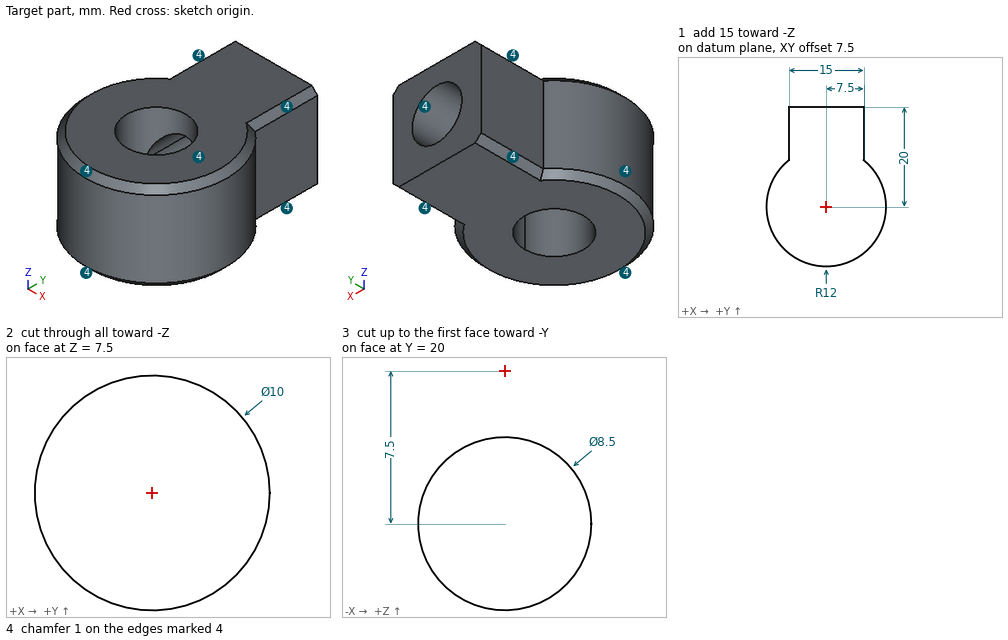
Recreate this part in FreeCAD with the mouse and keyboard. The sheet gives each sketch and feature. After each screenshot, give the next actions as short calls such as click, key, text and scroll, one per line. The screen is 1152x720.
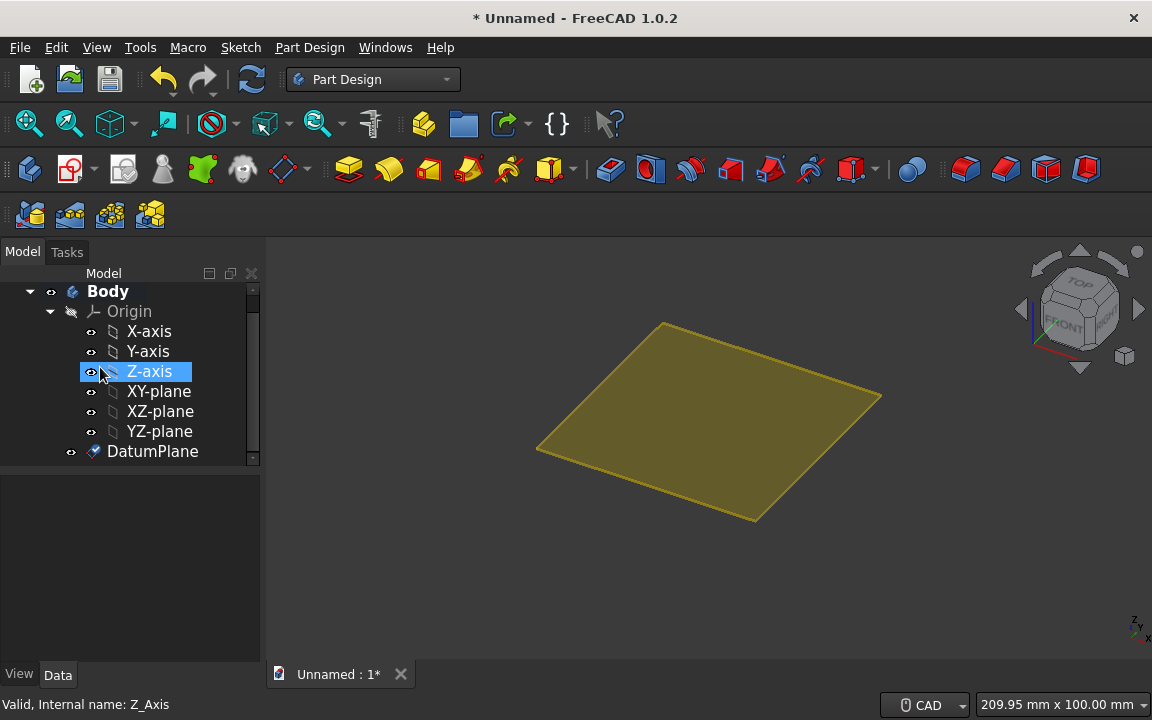
click(116, 452)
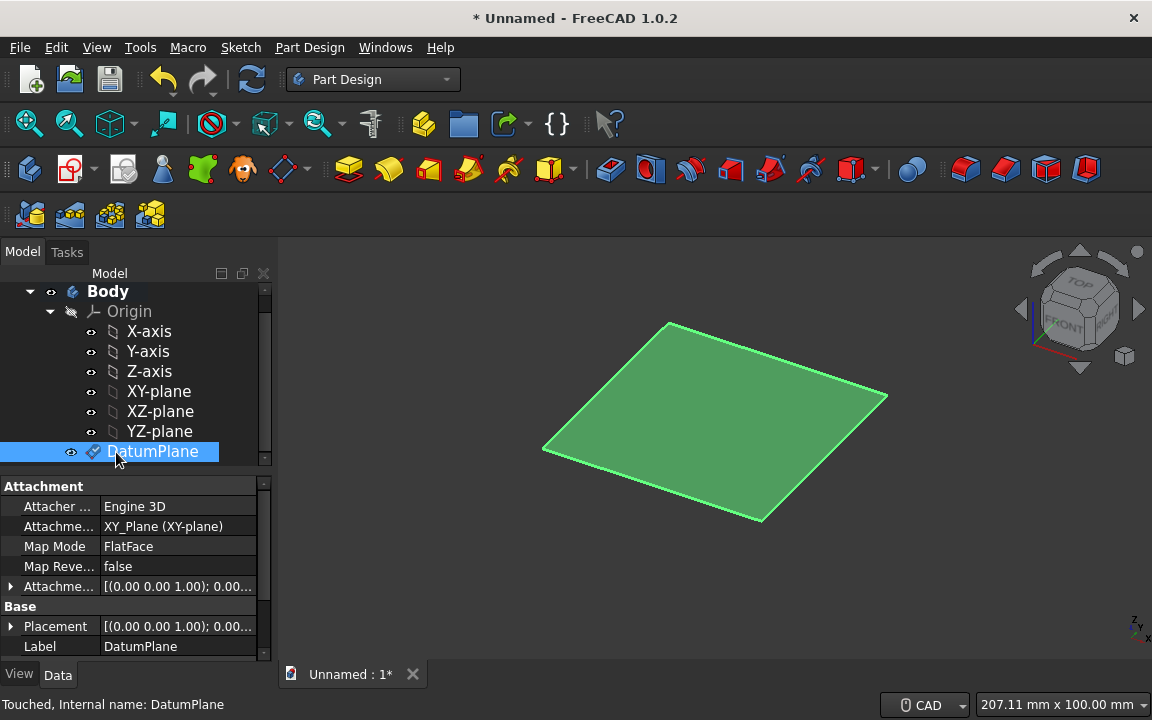
click(70, 170)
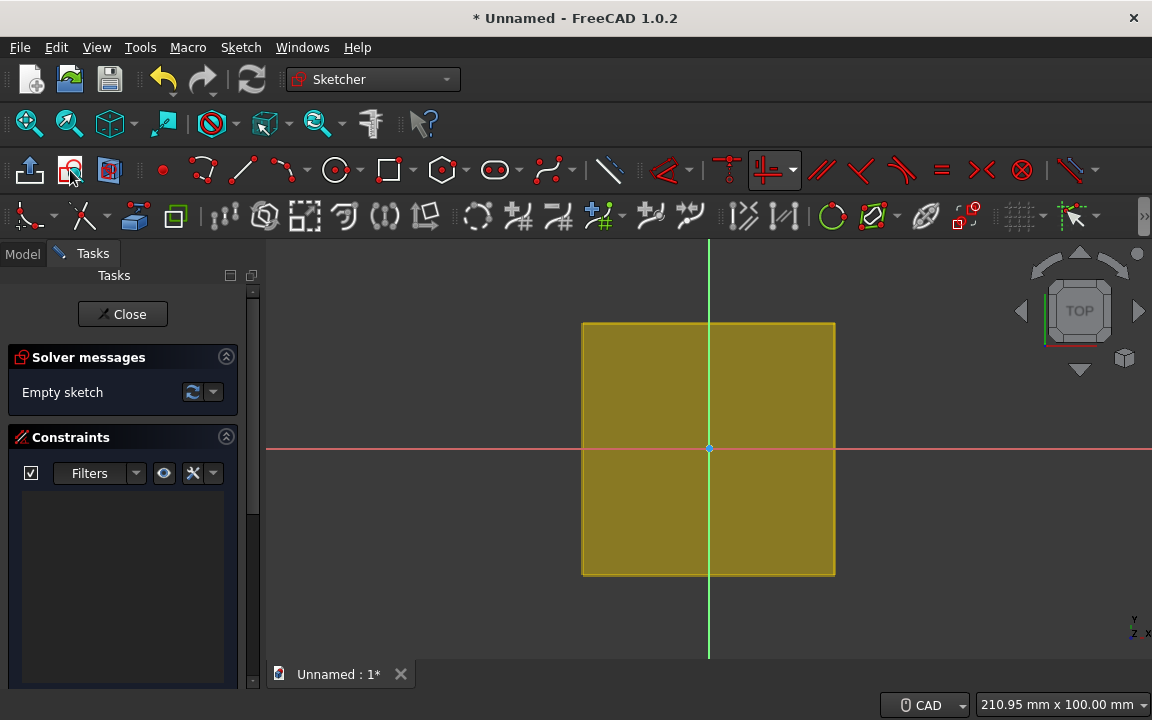
scroll(792, 412, up, 3)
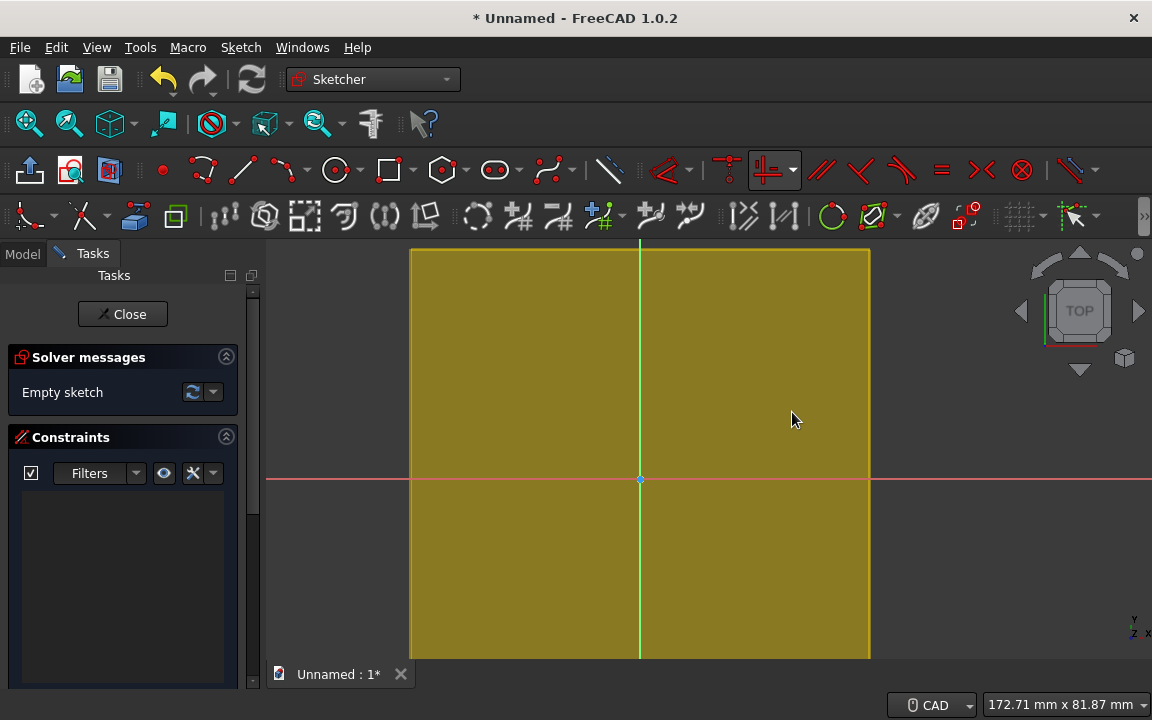
click(204, 170)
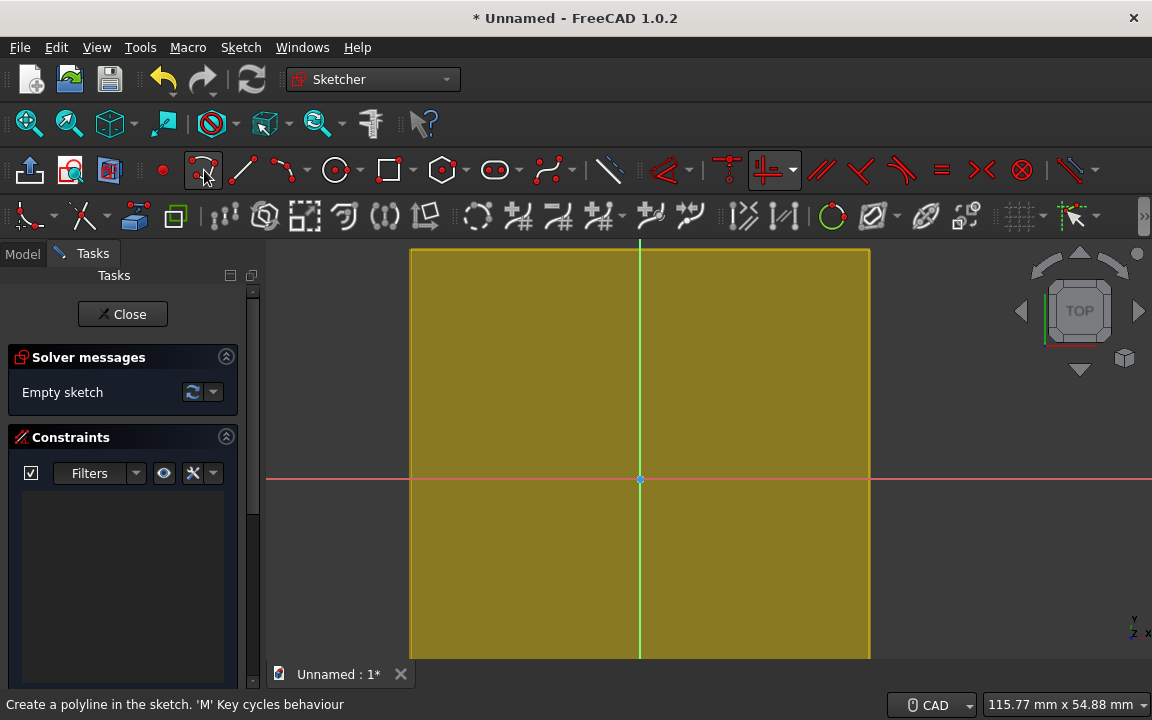
click(698, 407)
click(698, 326)
click(583, 326)
click(583, 407)
right_click(583, 407)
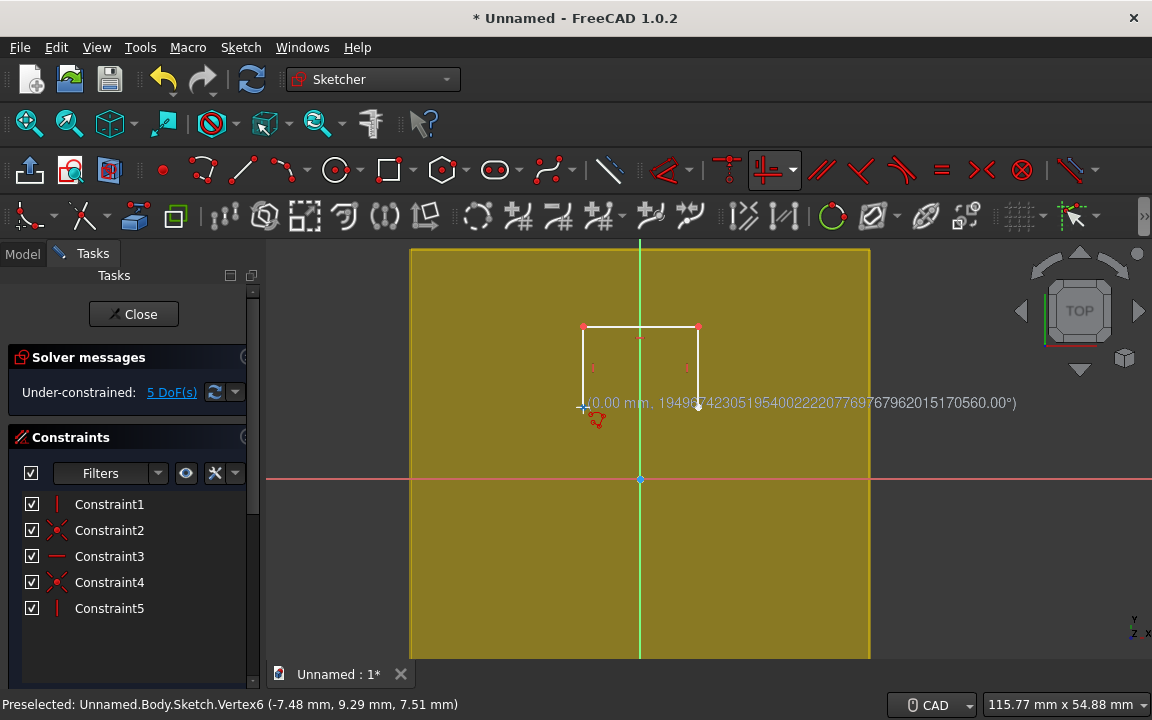
click(284, 170)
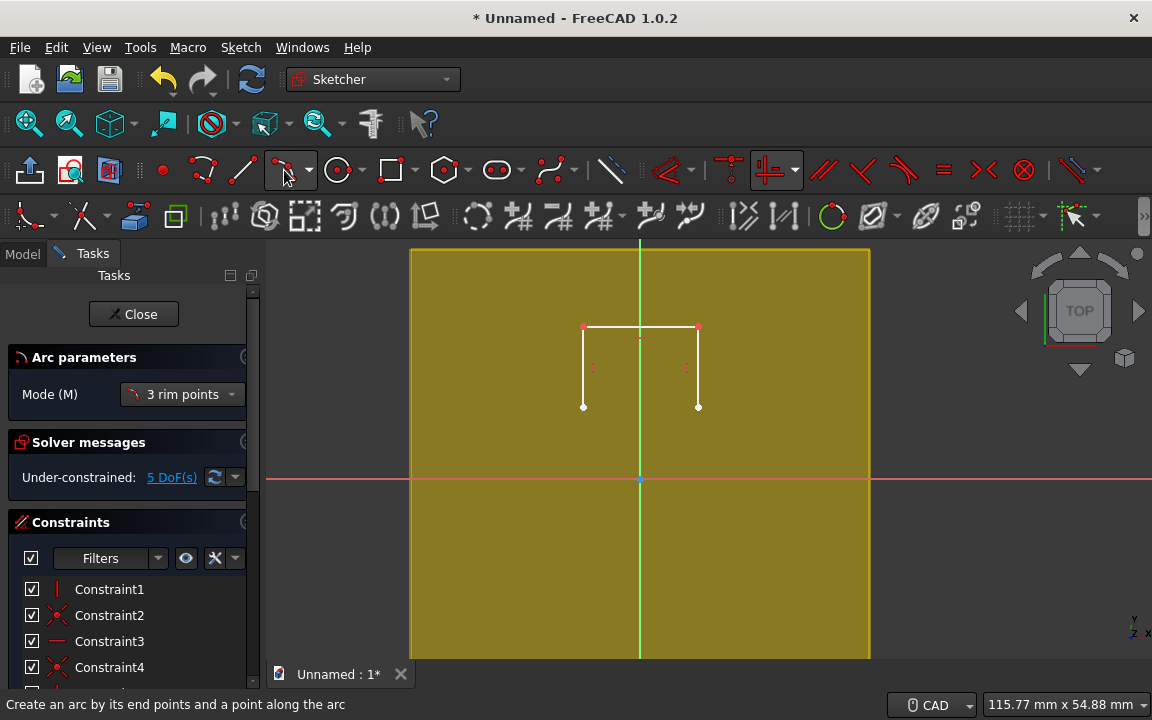
click(583, 408)
click(698, 408)
click(597, 560)
key(Escape)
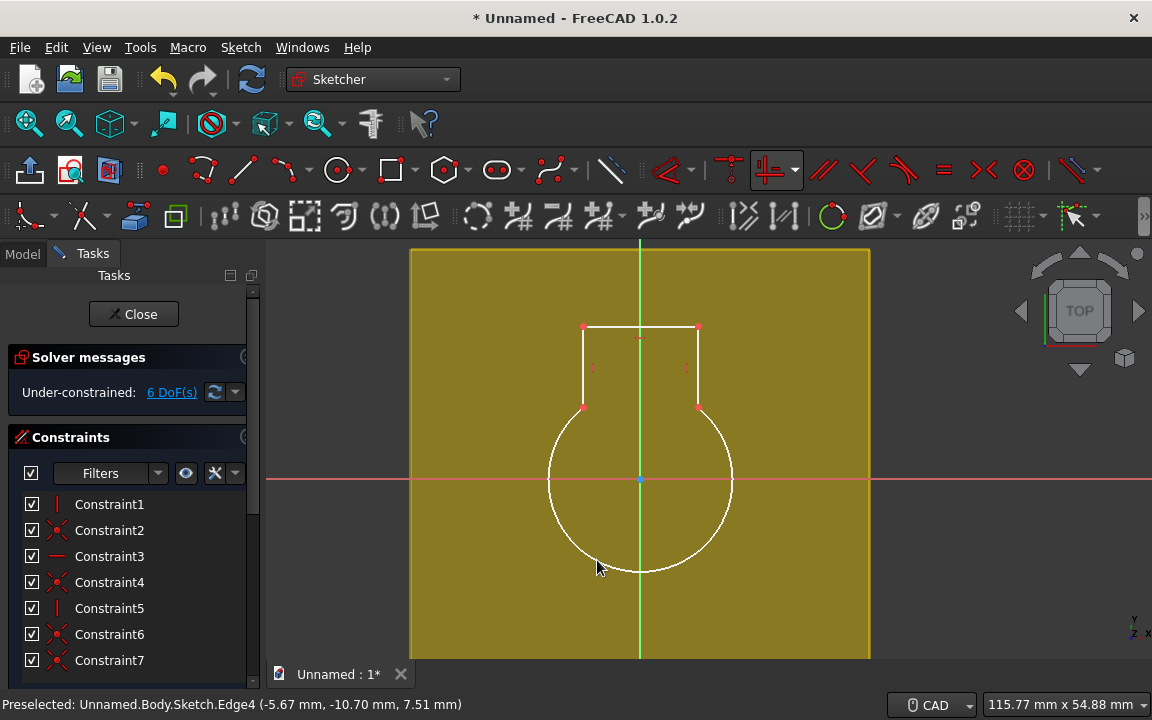
drag(630, 469, 651, 490)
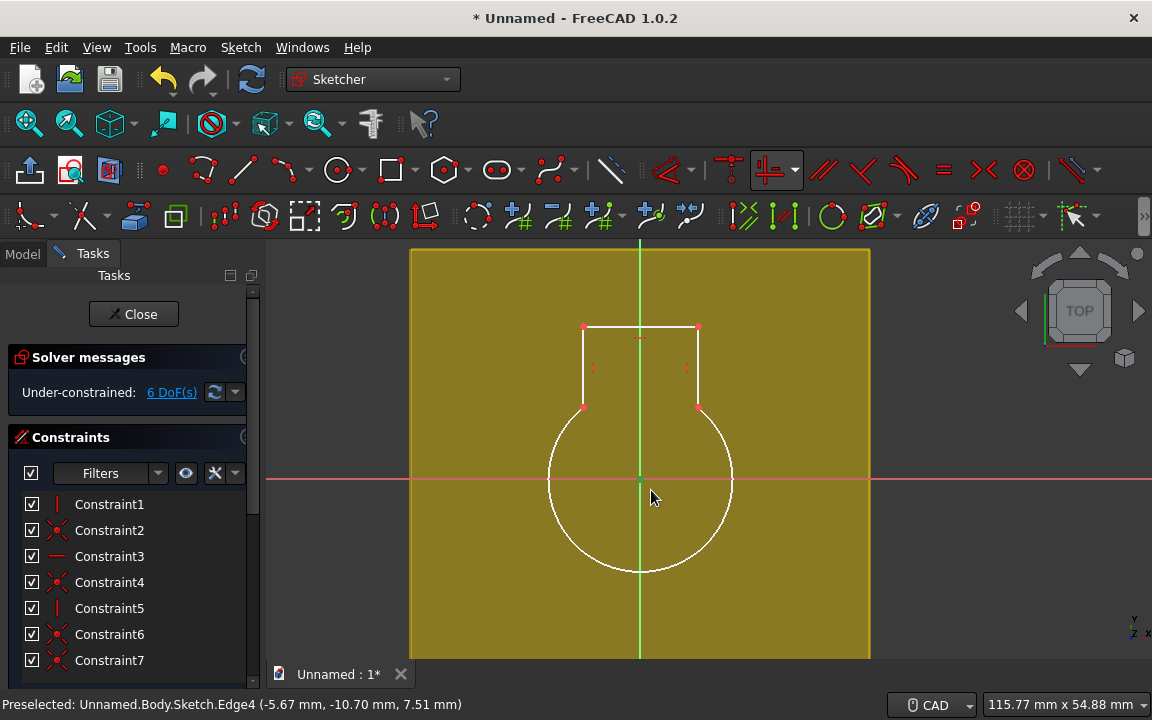
click(730, 170)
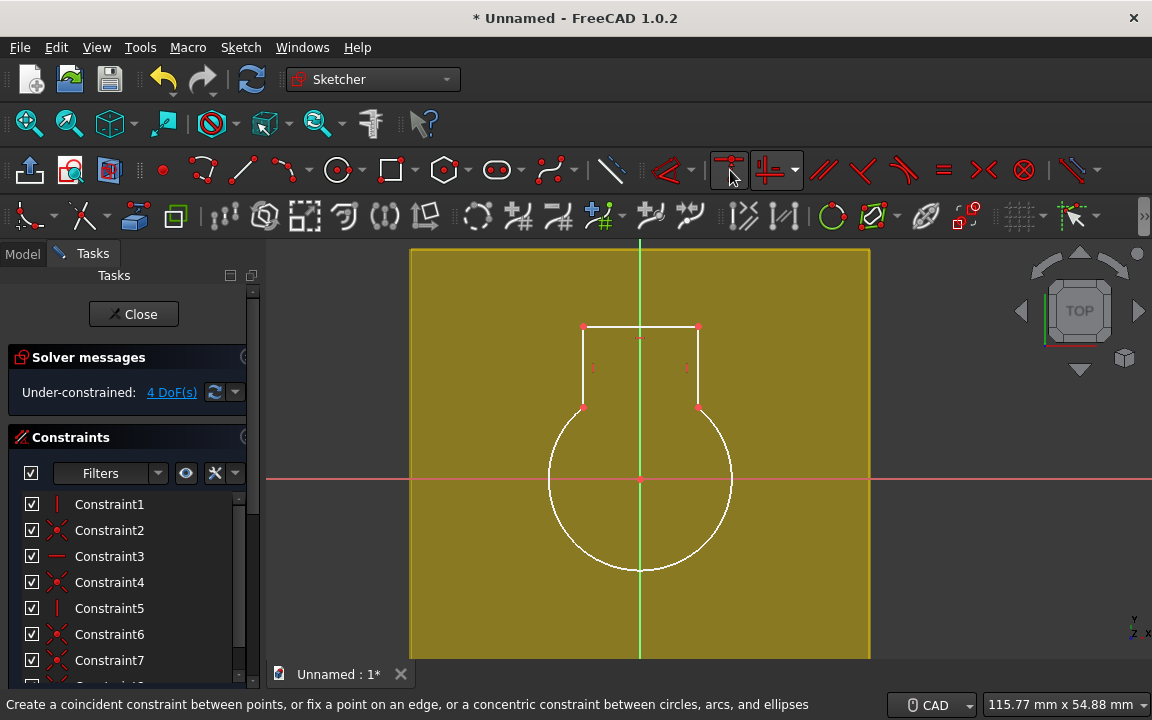
click(666, 170)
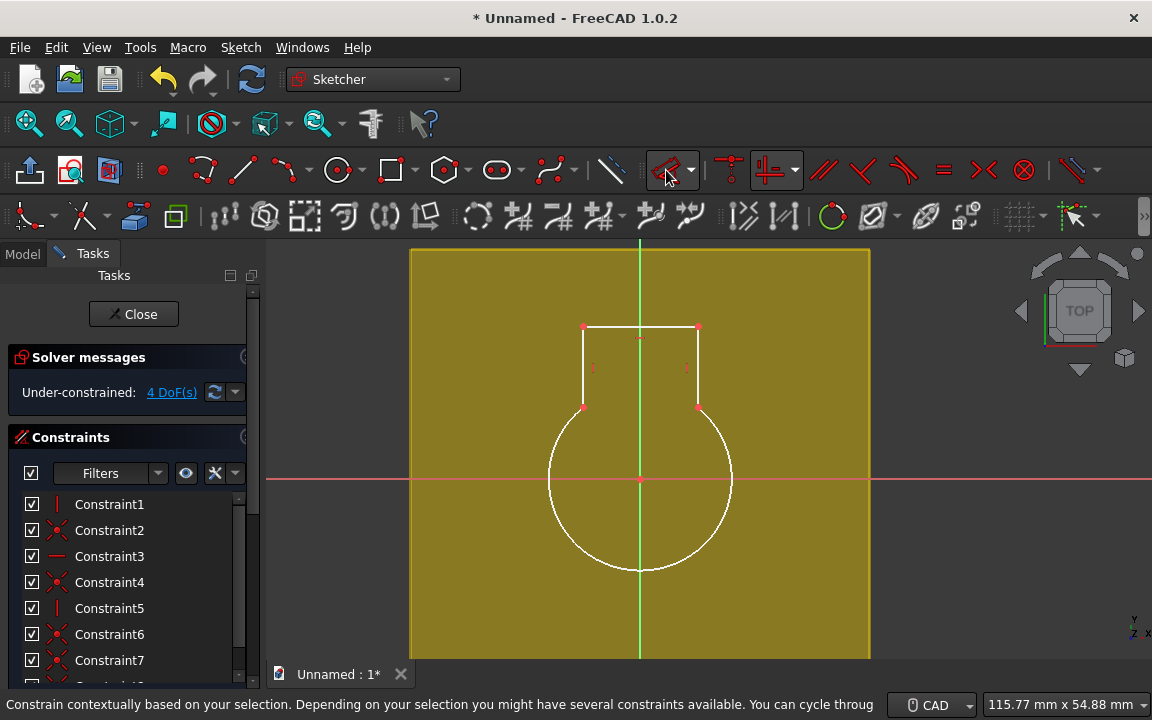
click(564, 529)
click(537, 547)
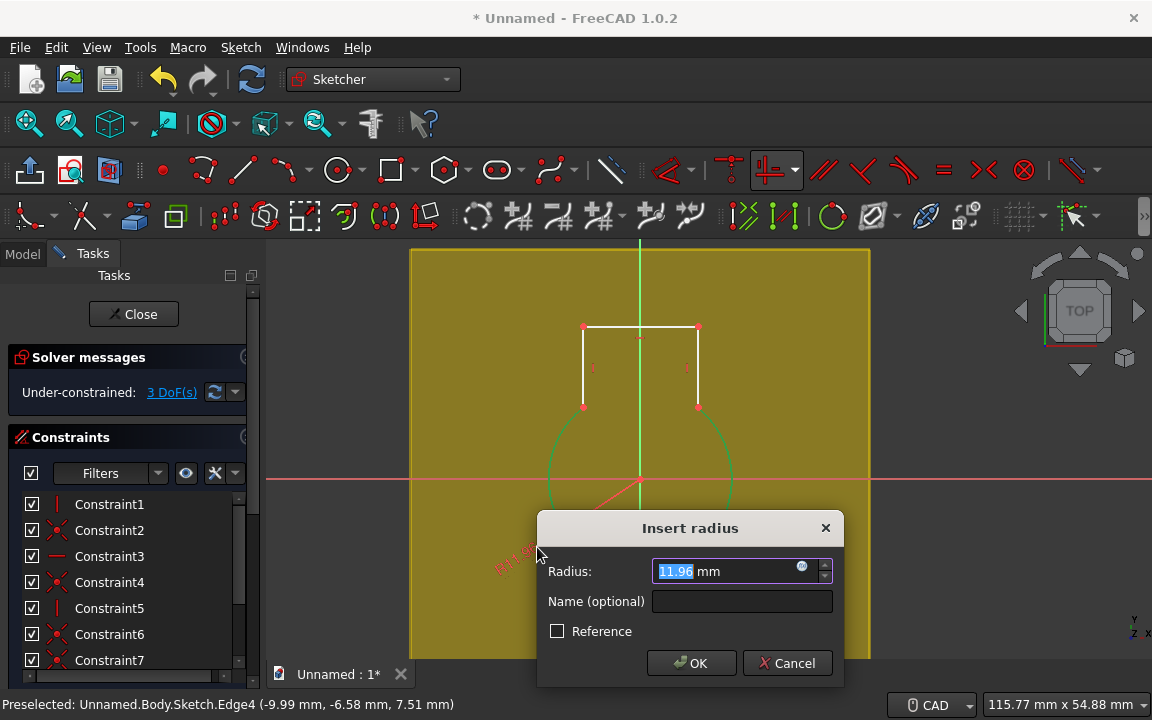
text(12)
key(Return)